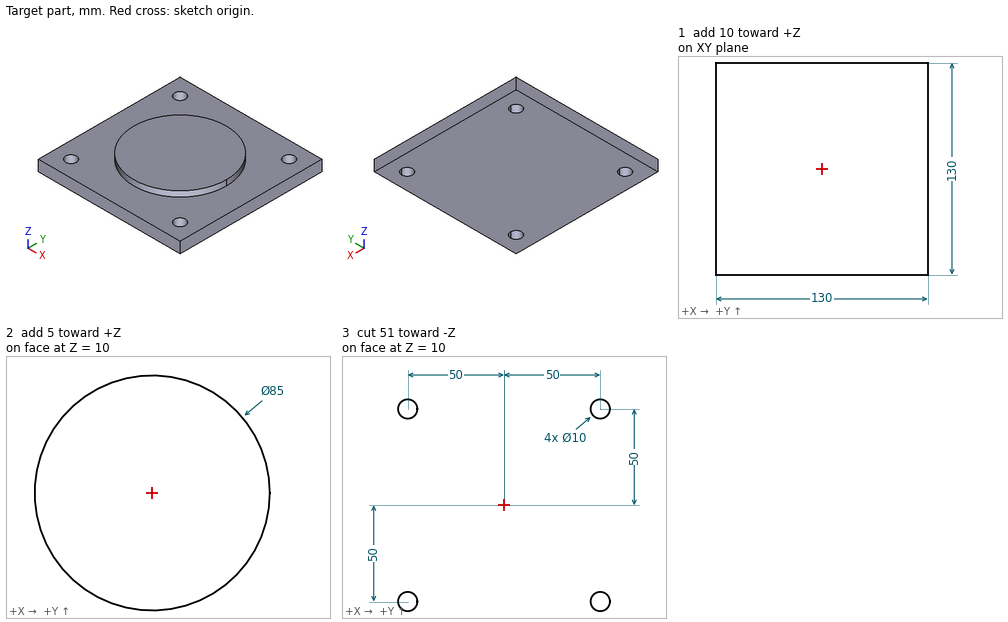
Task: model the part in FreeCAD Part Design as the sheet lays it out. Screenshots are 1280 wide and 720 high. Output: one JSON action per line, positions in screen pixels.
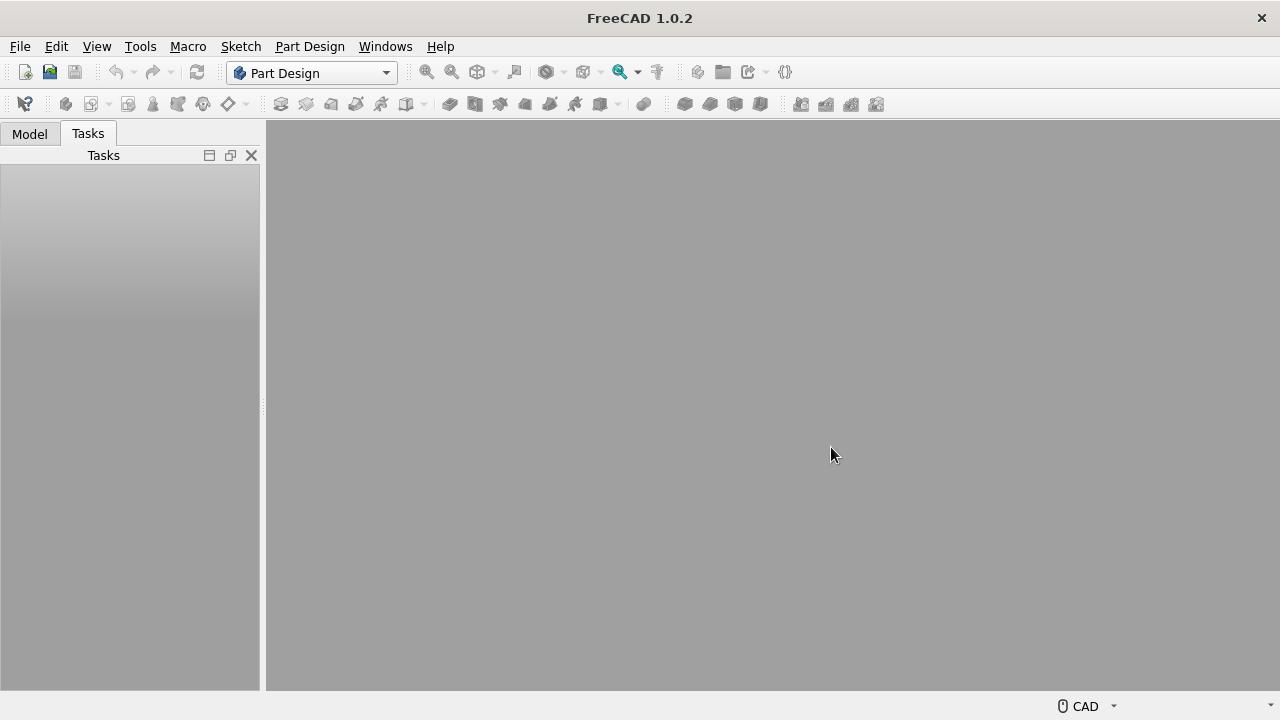
{"action": "left_click", "coordinate": [25, 72]}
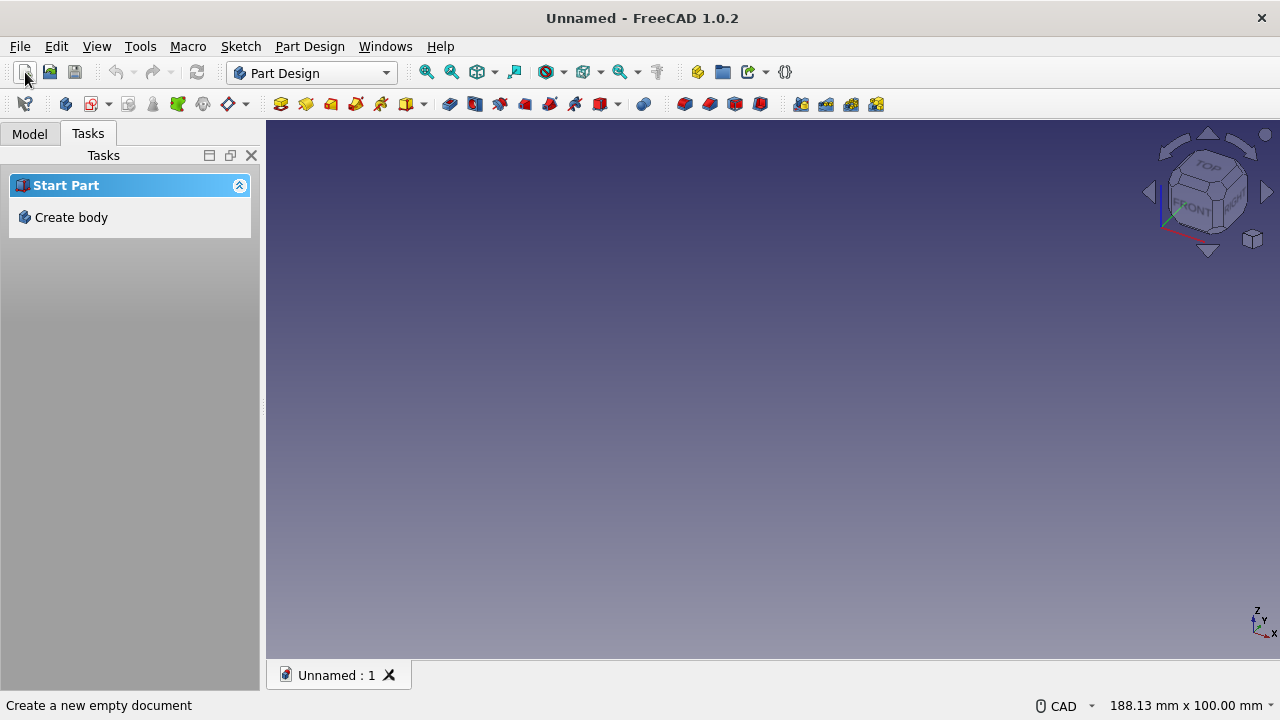
{"action": "left_click", "coordinate": [90, 104]}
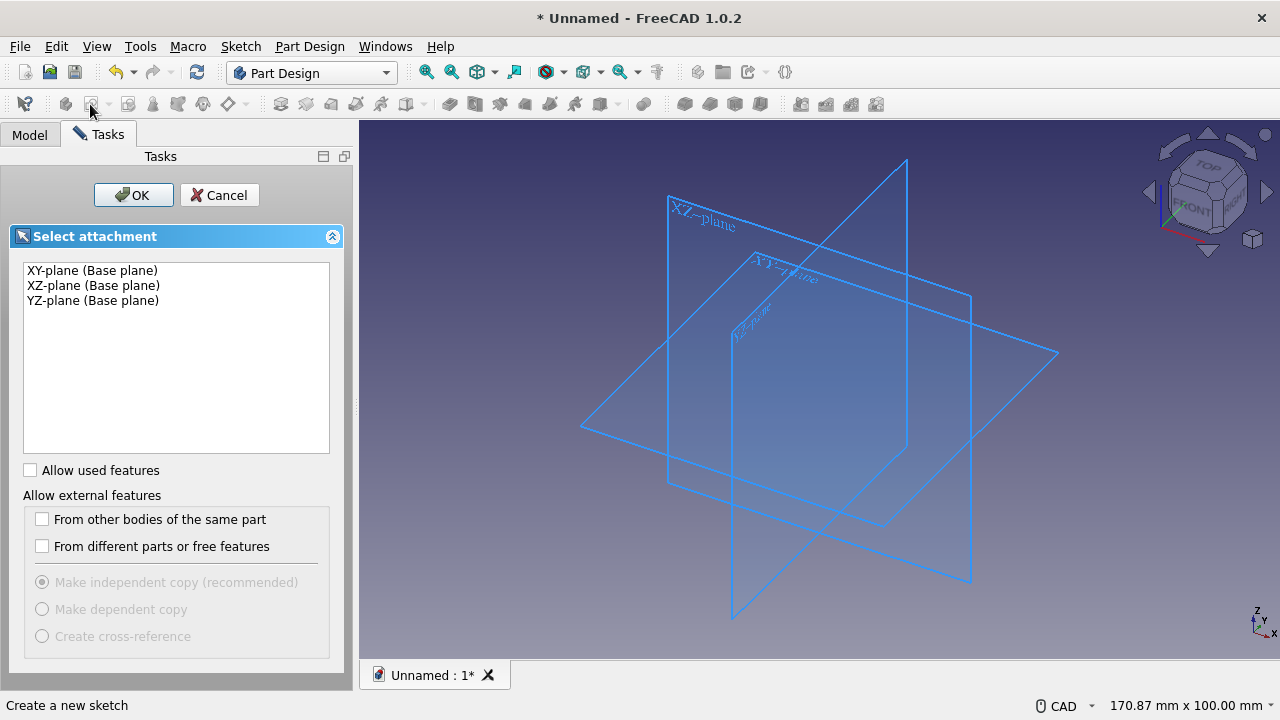
{"action": "left_click", "coordinate": [84, 270]}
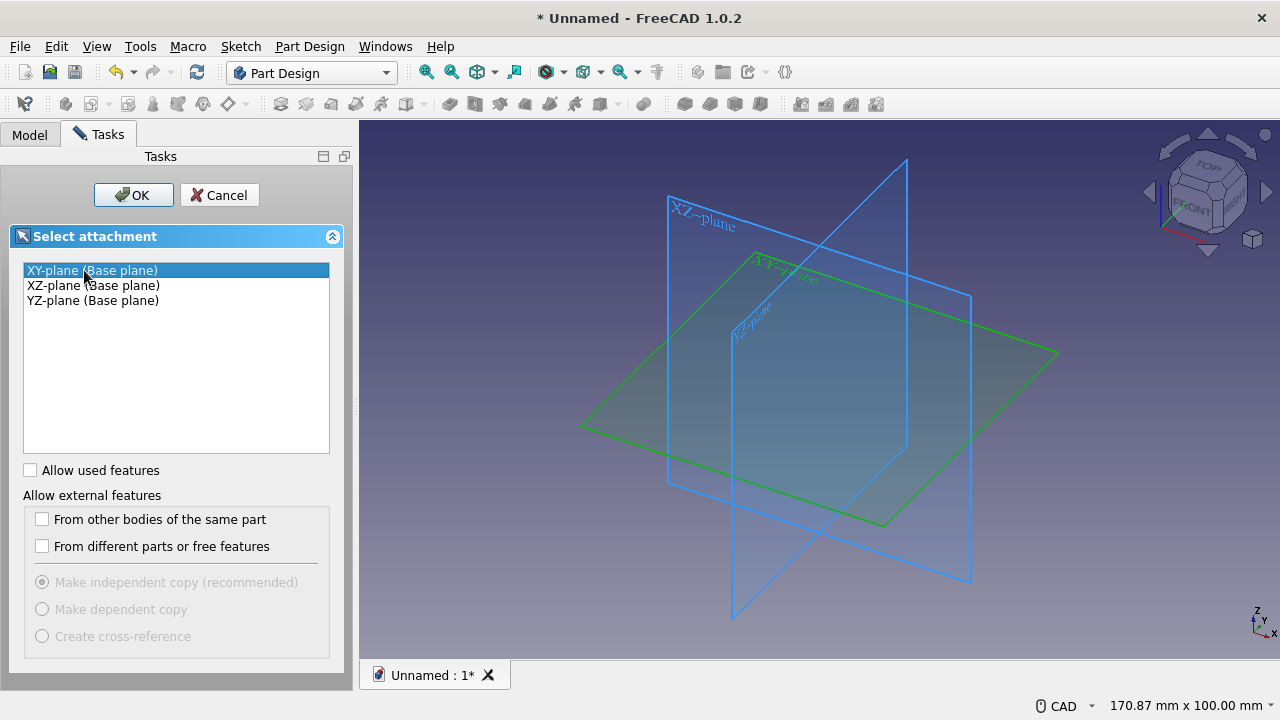
{"action": "left_click", "coordinate": [134, 195]}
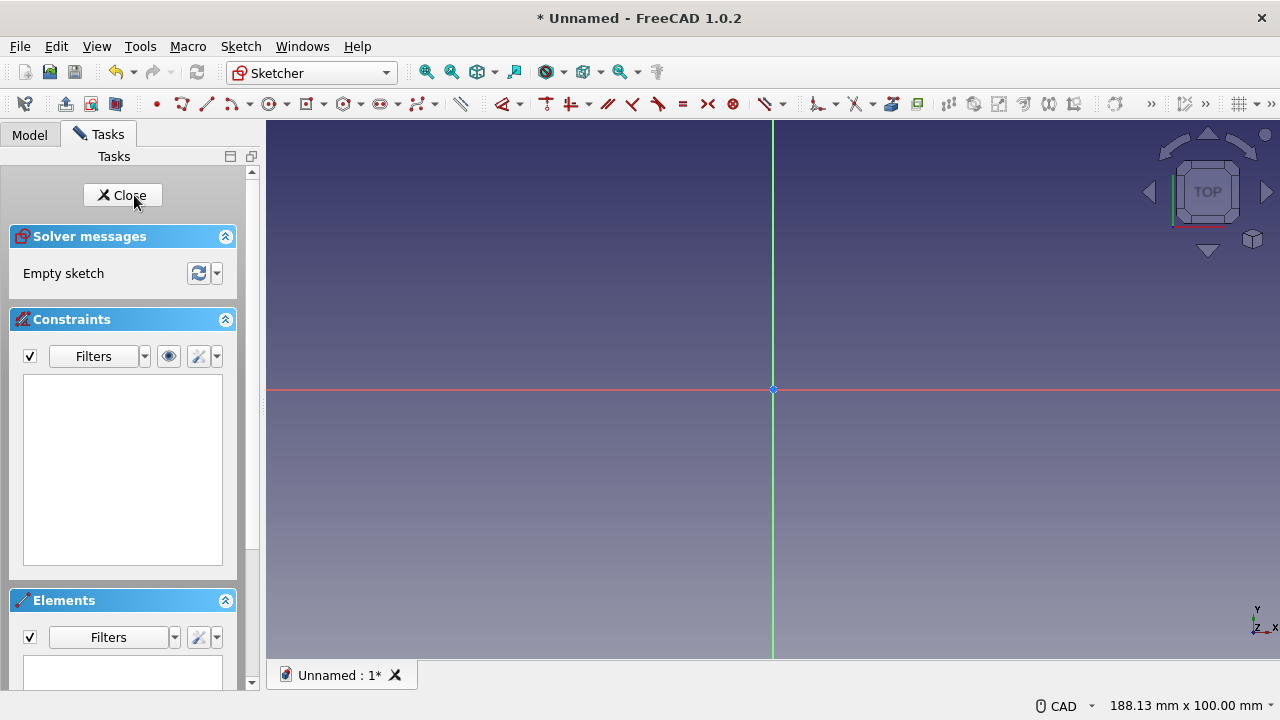
{"action": "scroll", "coordinate": [649, 390], "scroll_direction": "down", "scroll_amount": 4}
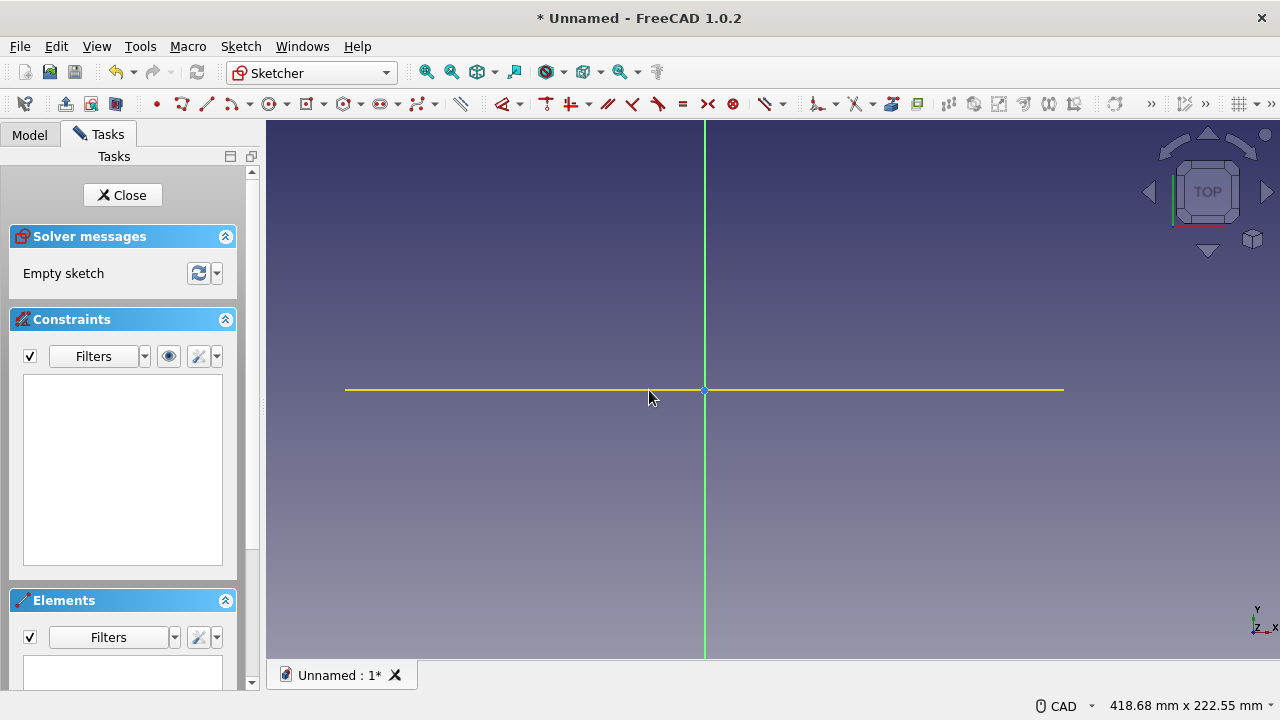
{"action": "left_click", "coordinate": [306, 104]}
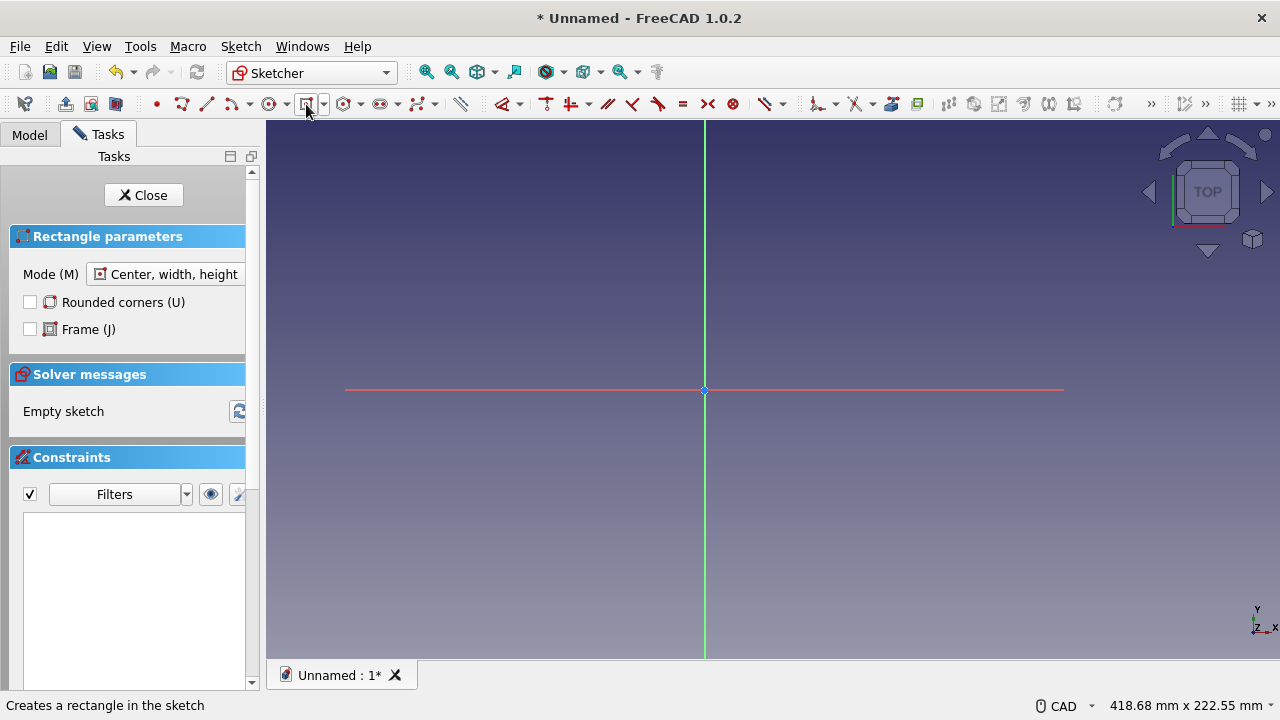
{"action": "left_click", "coordinate": [705, 390]}
{"action": "left_click", "coordinate": [862, 233]}
{"action": "key", "text": "Escape"}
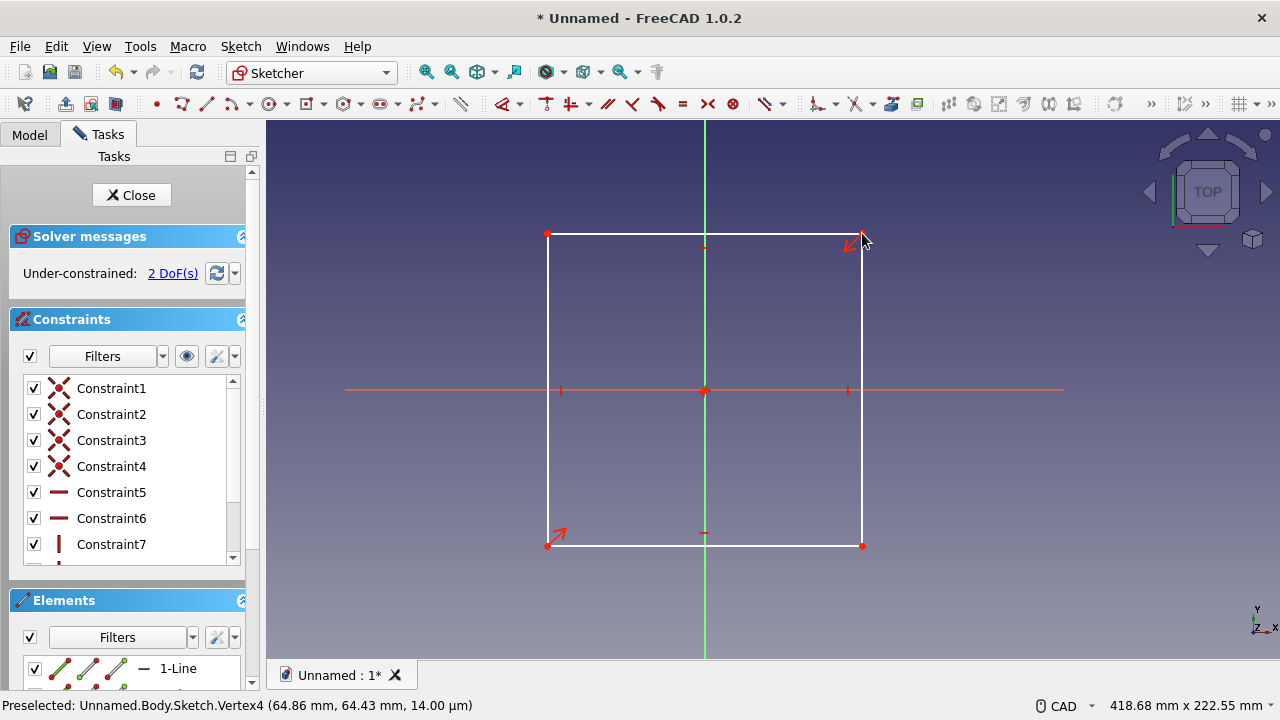
{"action": "left_click", "coordinate": [642, 546]}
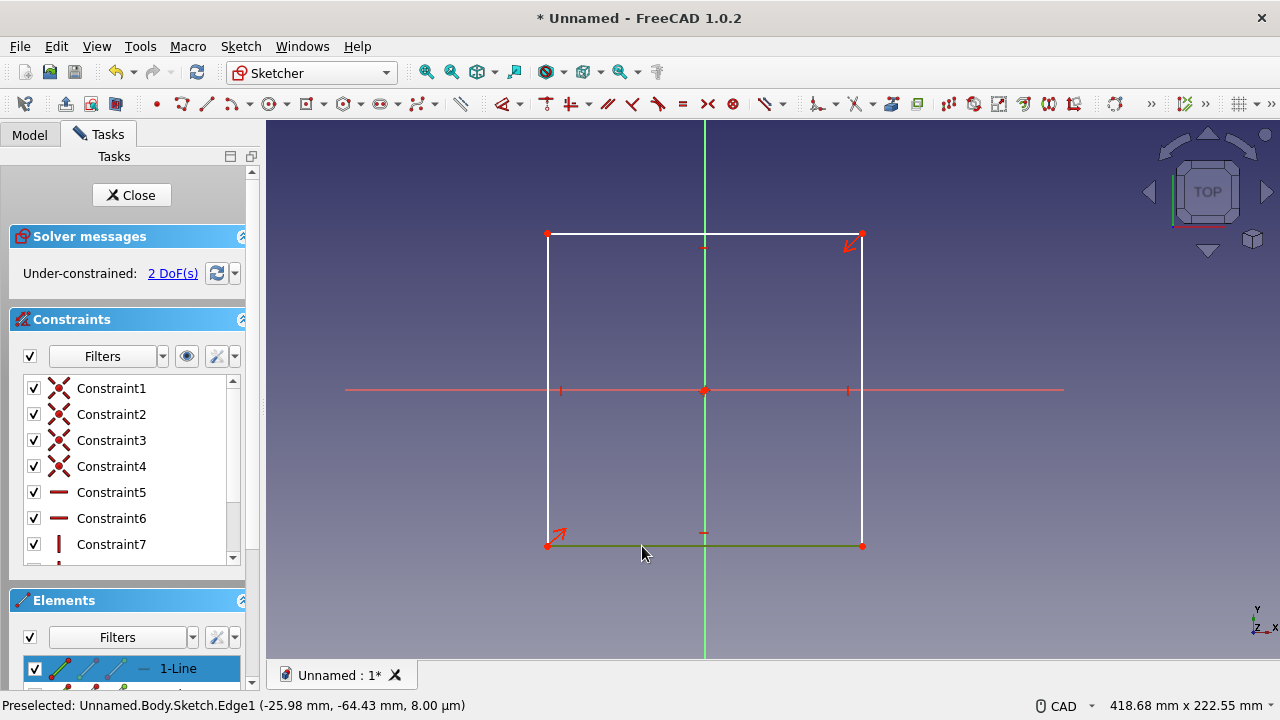
{"action": "left_click", "coordinate": [520, 104]}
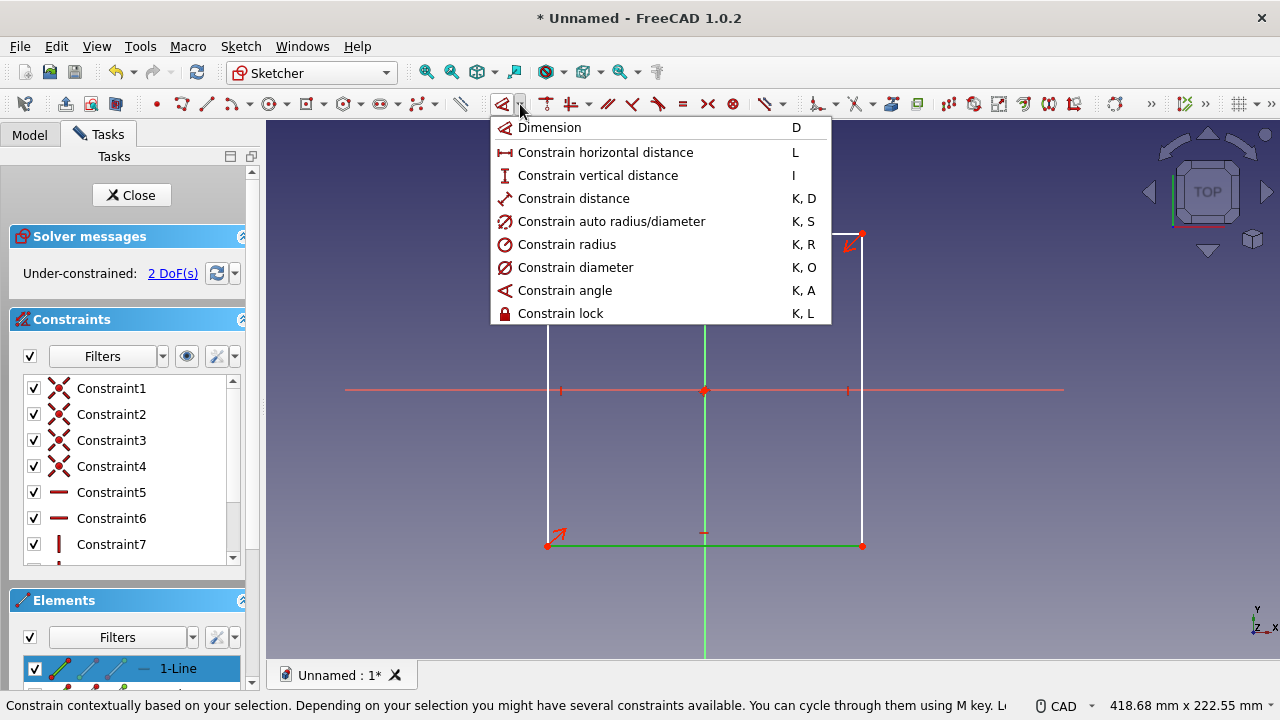
{"action": "left_click", "coordinate": [661, 152]}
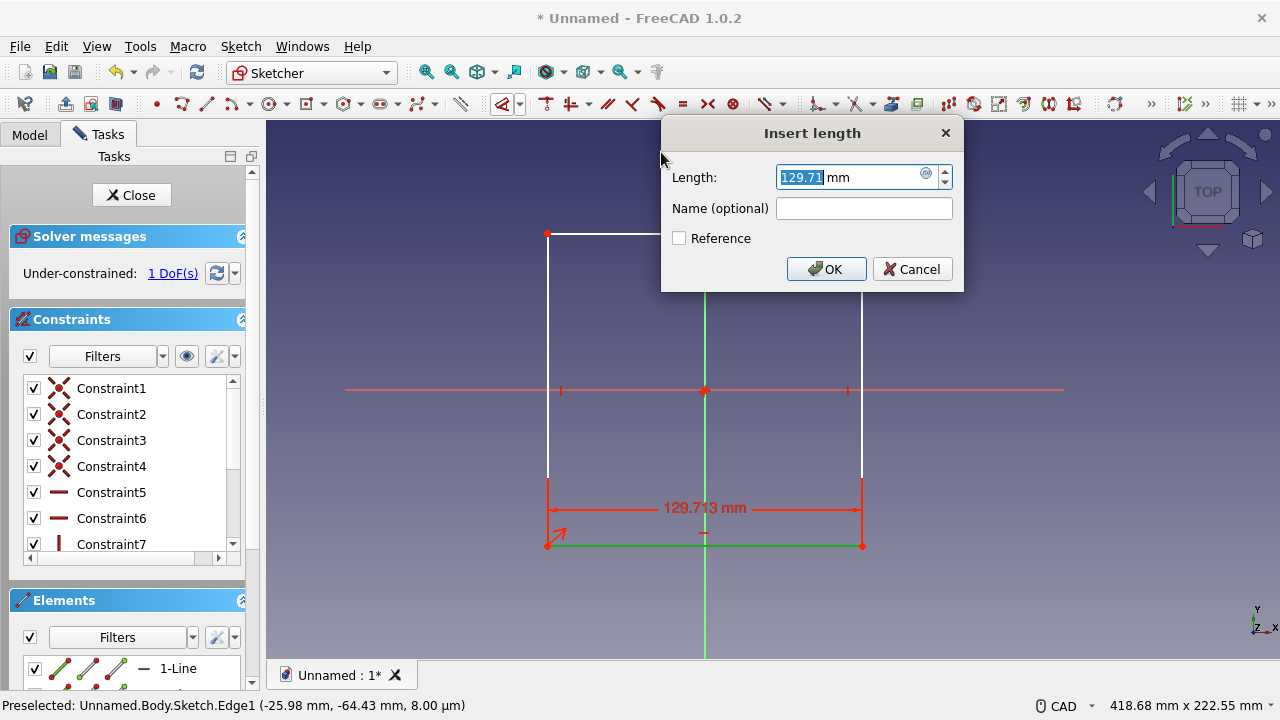
{"action": "type", "text": "130"}
{"action": "key", "text": "Return"}